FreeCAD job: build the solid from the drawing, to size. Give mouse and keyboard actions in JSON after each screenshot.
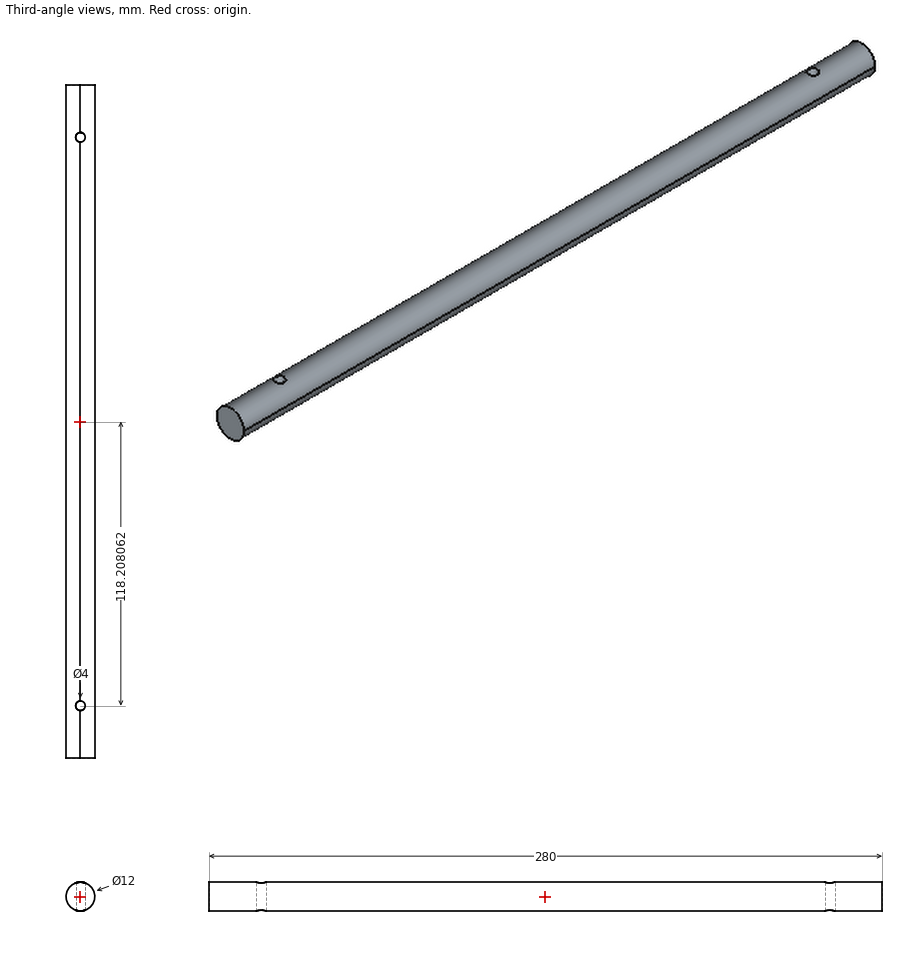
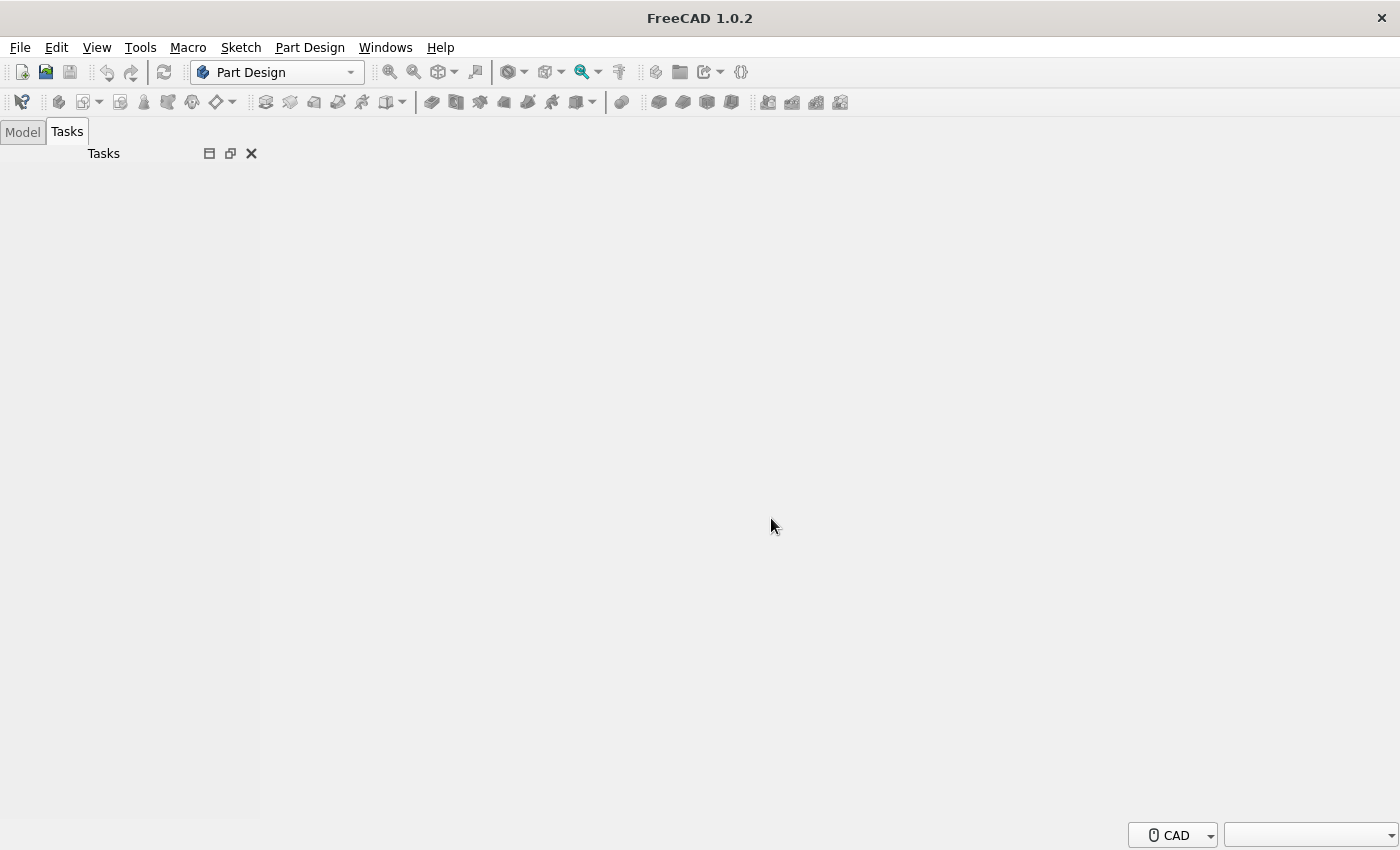
{"action": "left_click", "coordinate": [22, 72]}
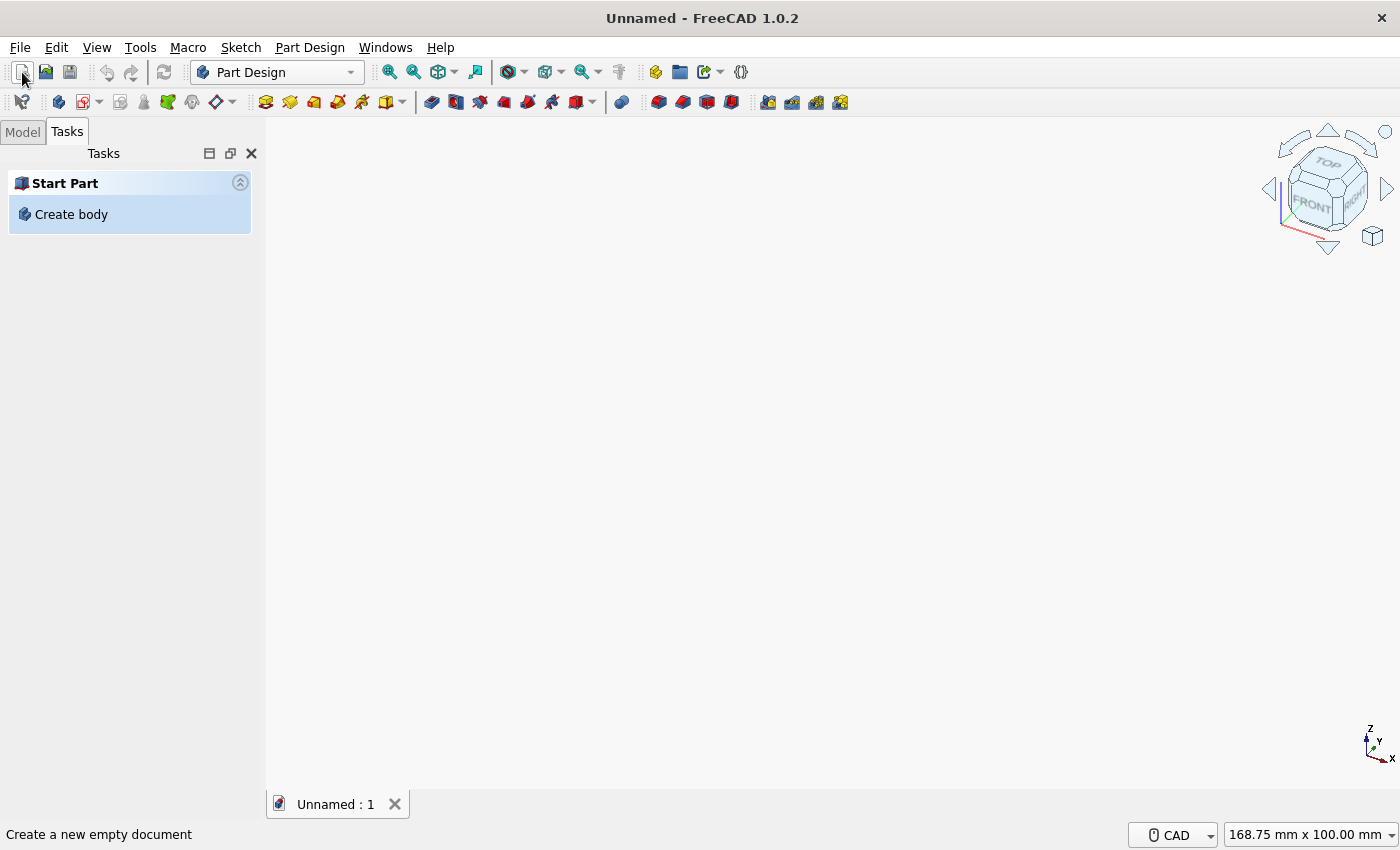
{"action": "left_click", "coordinate": [84, 102]}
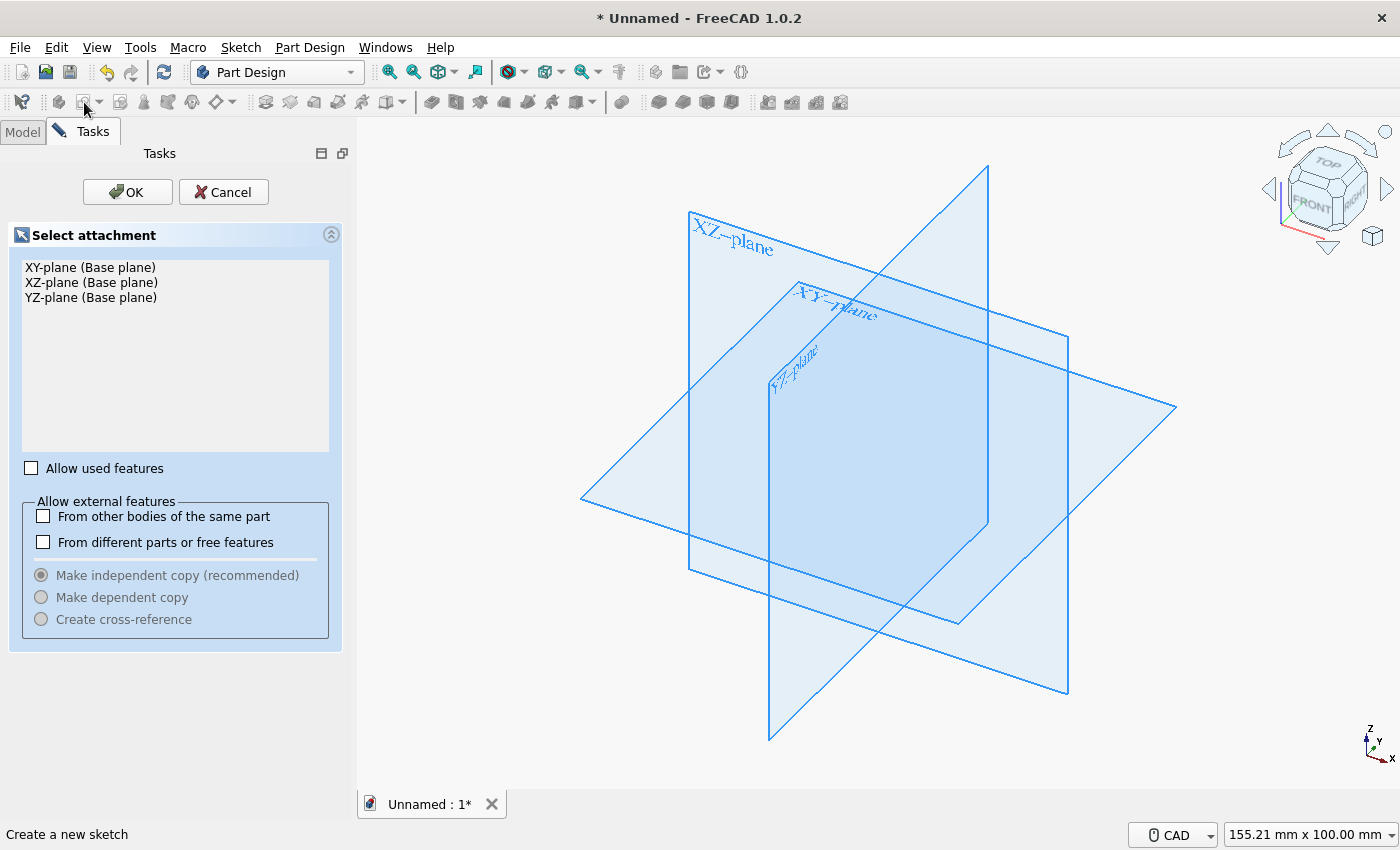
{"action": "left_click", "coordinate": [82, 282]}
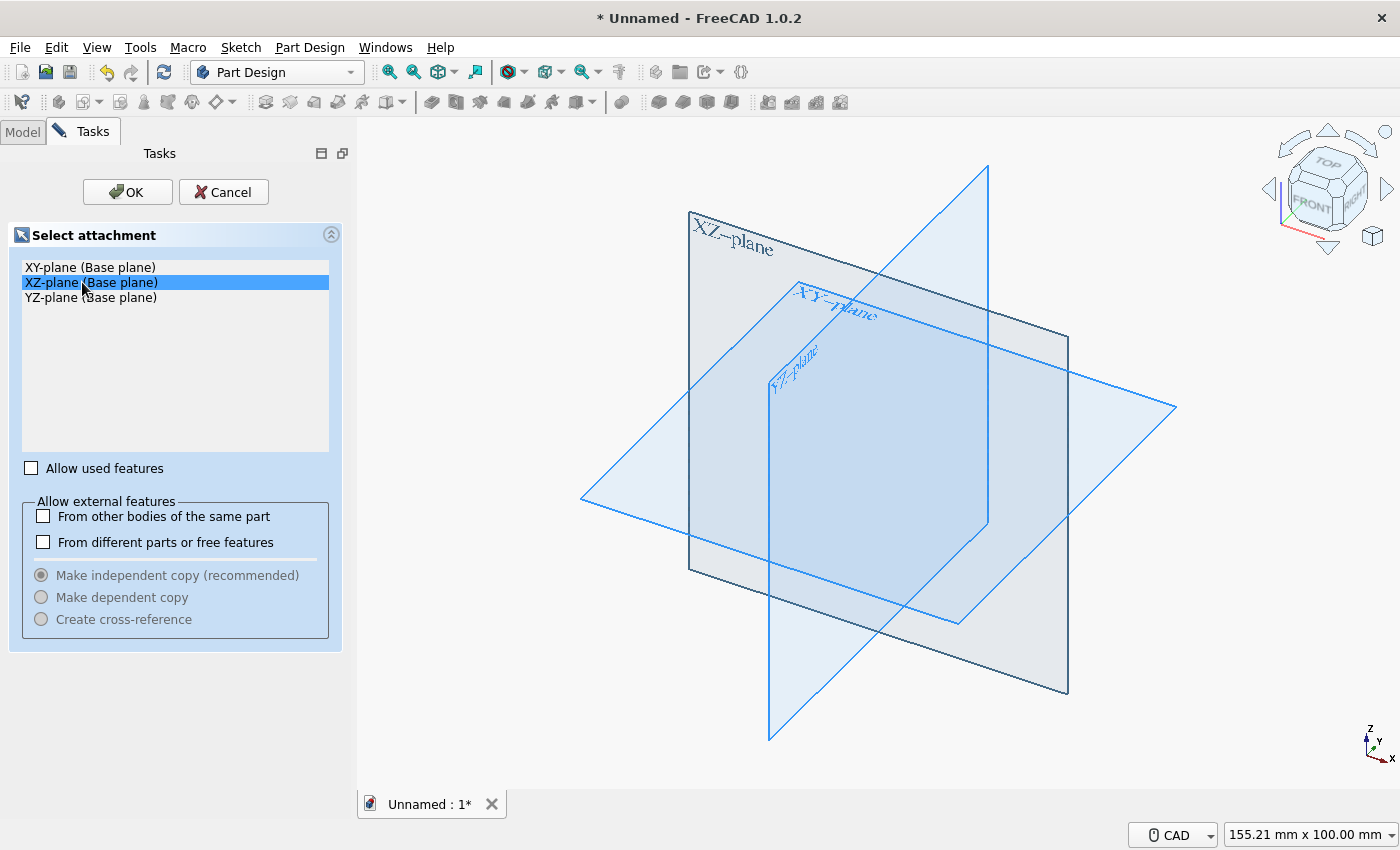
{"action": "left_click", "coordinate": [128, 192]}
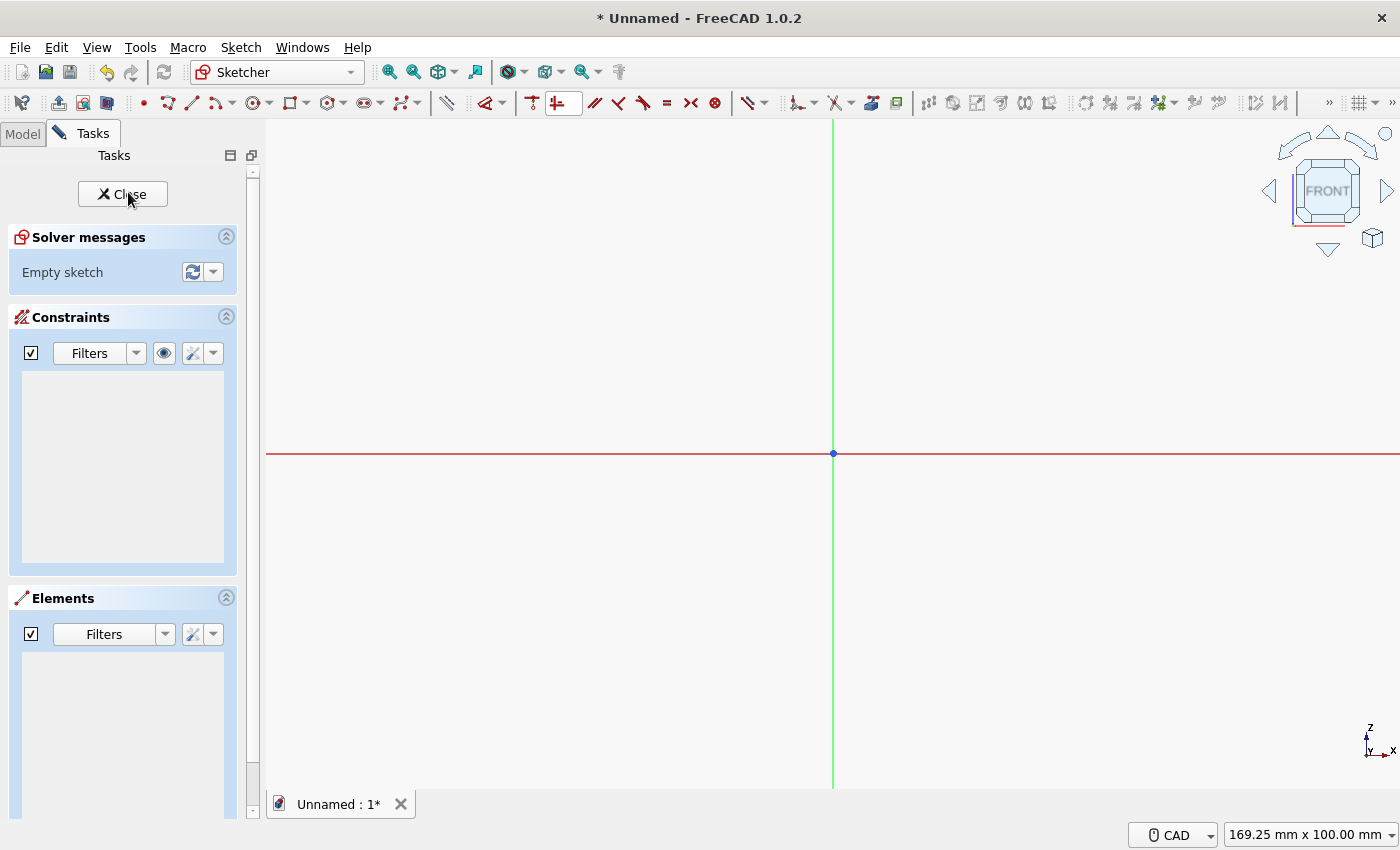
{"action": "scroll", "coordinate": [850, 454], "scroll_direction": "up", "scroll_amount": 8}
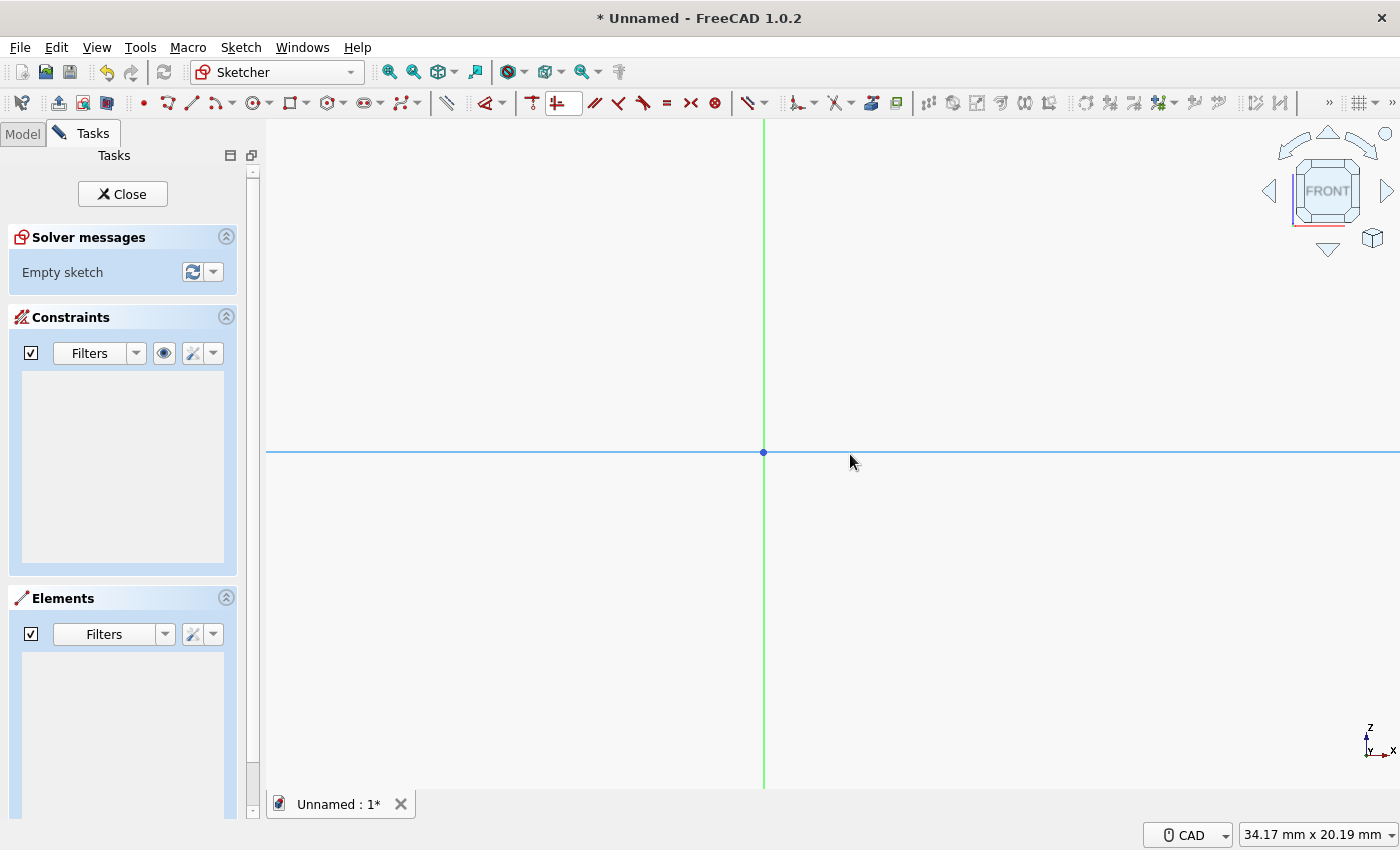
{"action": "left_click", "coordinate": [254, 104]}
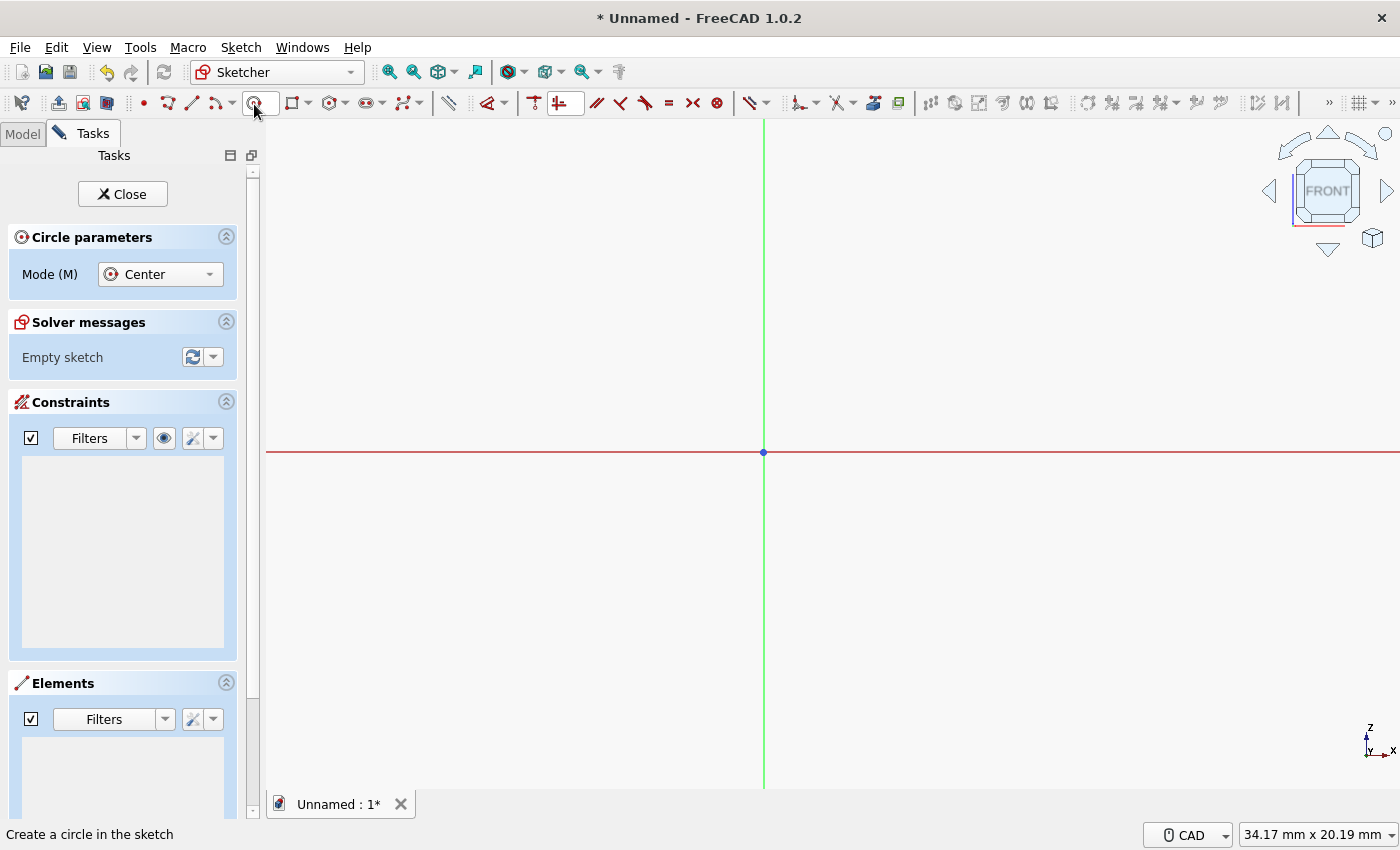
{"action": "left_click", "coordinate": [764, 452]}
{"action": "left_click", "coordinate": [905, 311]}
{"action": "key", "text": "Escape"}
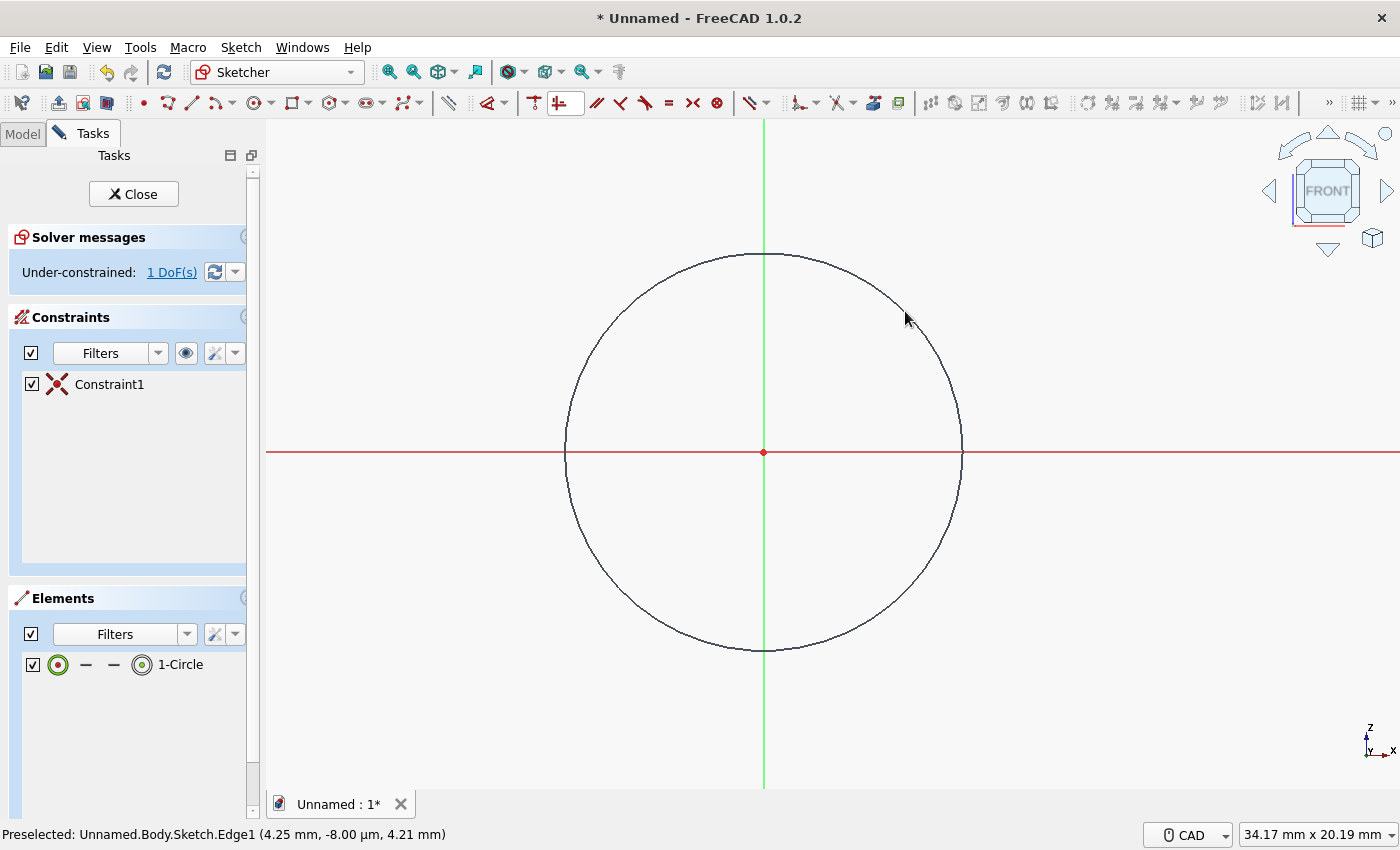
{"action": "left_click", "coordinate": [904, 311]}